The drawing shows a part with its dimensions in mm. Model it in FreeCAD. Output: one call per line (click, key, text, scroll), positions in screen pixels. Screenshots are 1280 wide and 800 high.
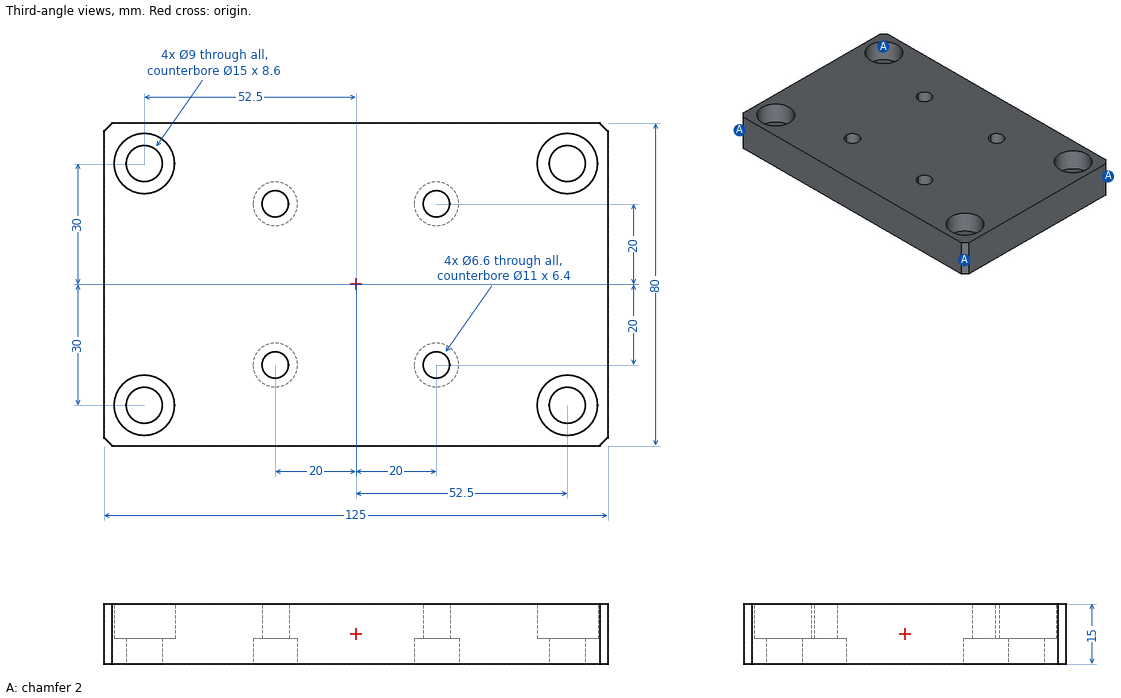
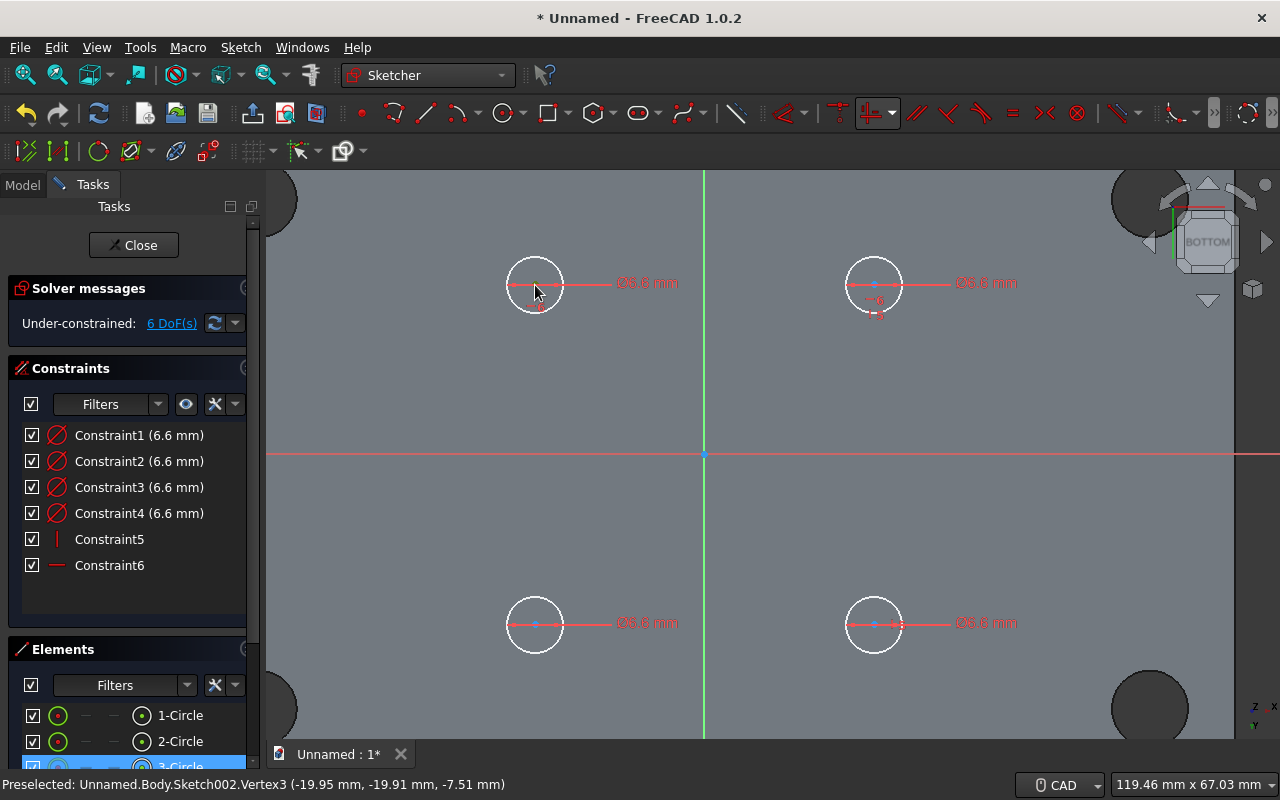
click(535, 625)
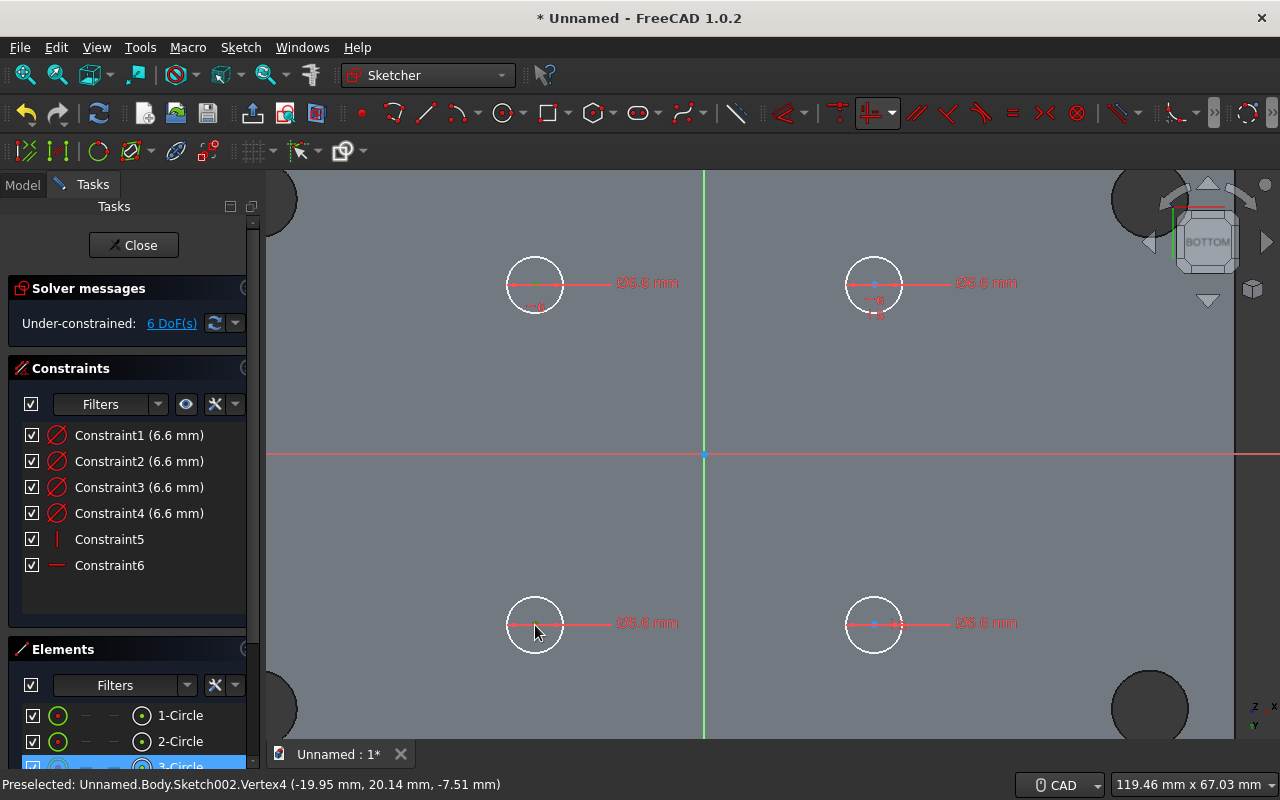
click(894, 114)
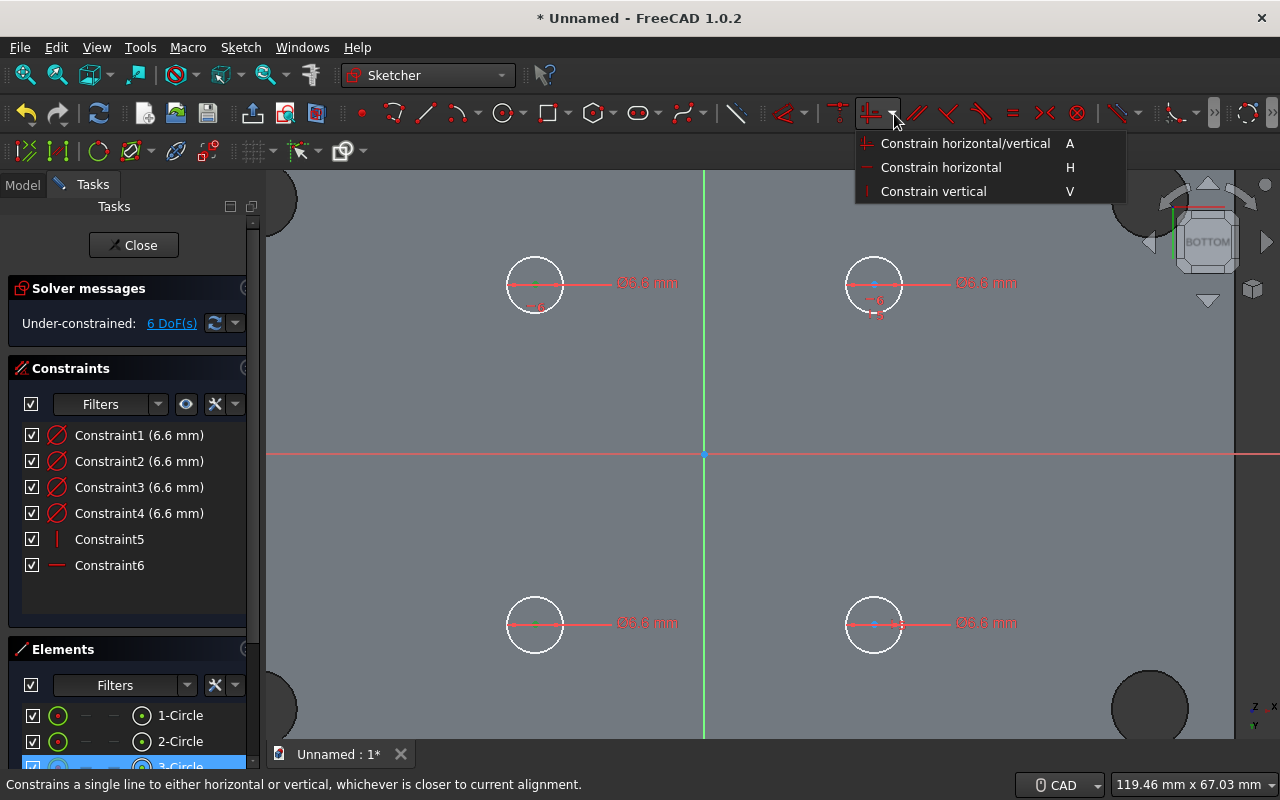
click(991, 191)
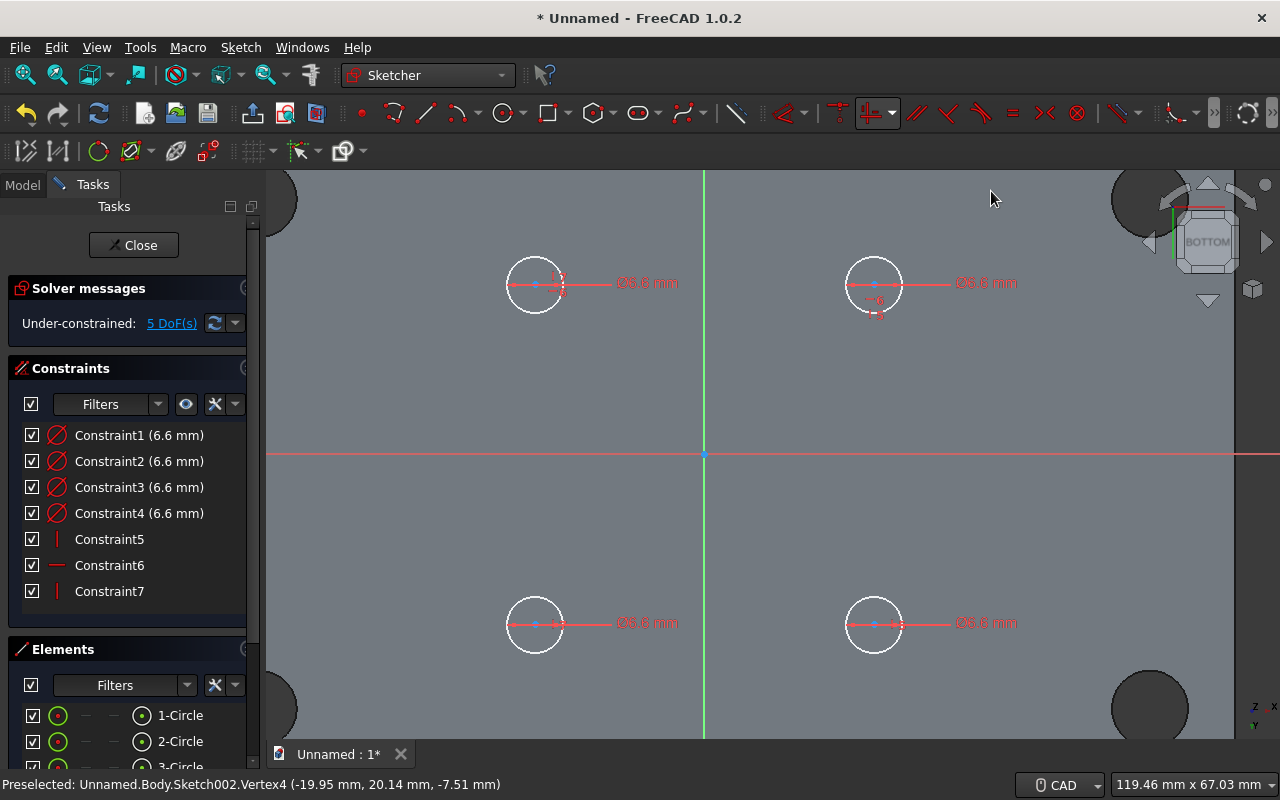
click(874, 625)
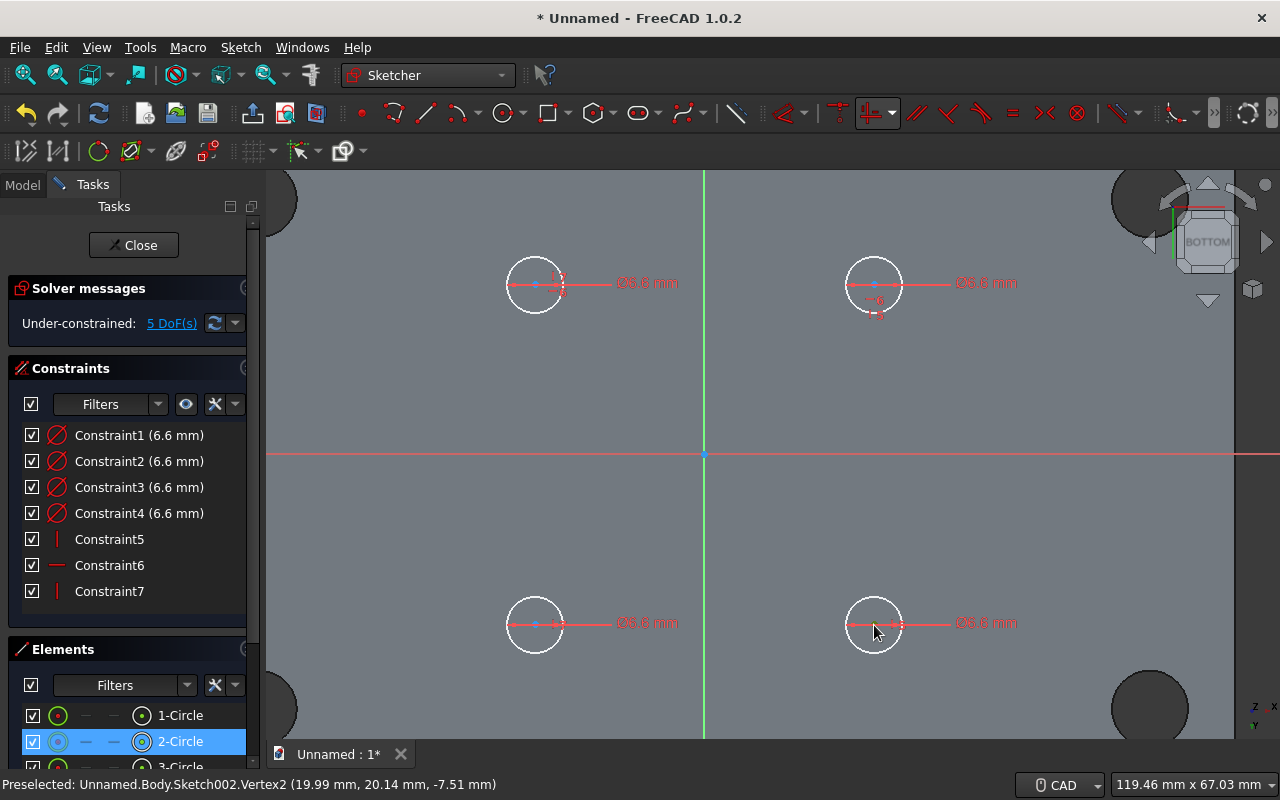
click(535, 625)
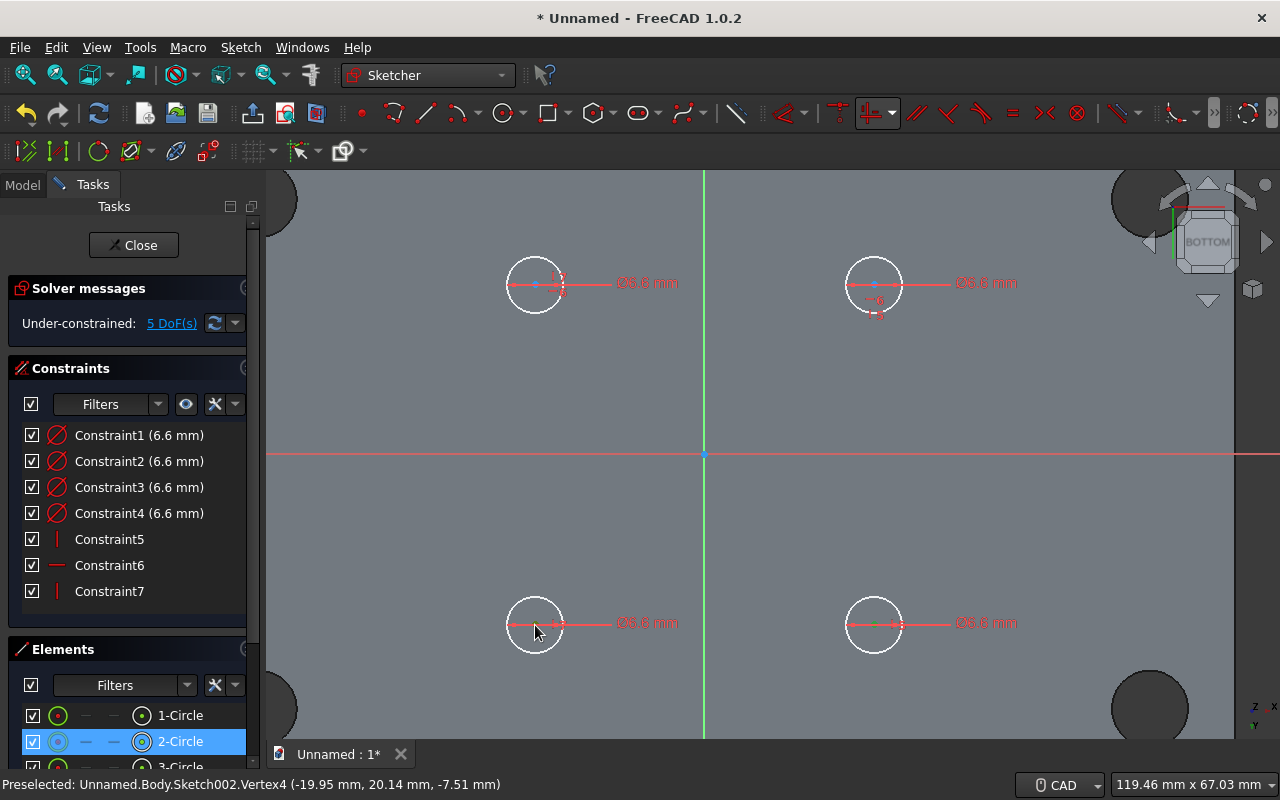
click(894, 114)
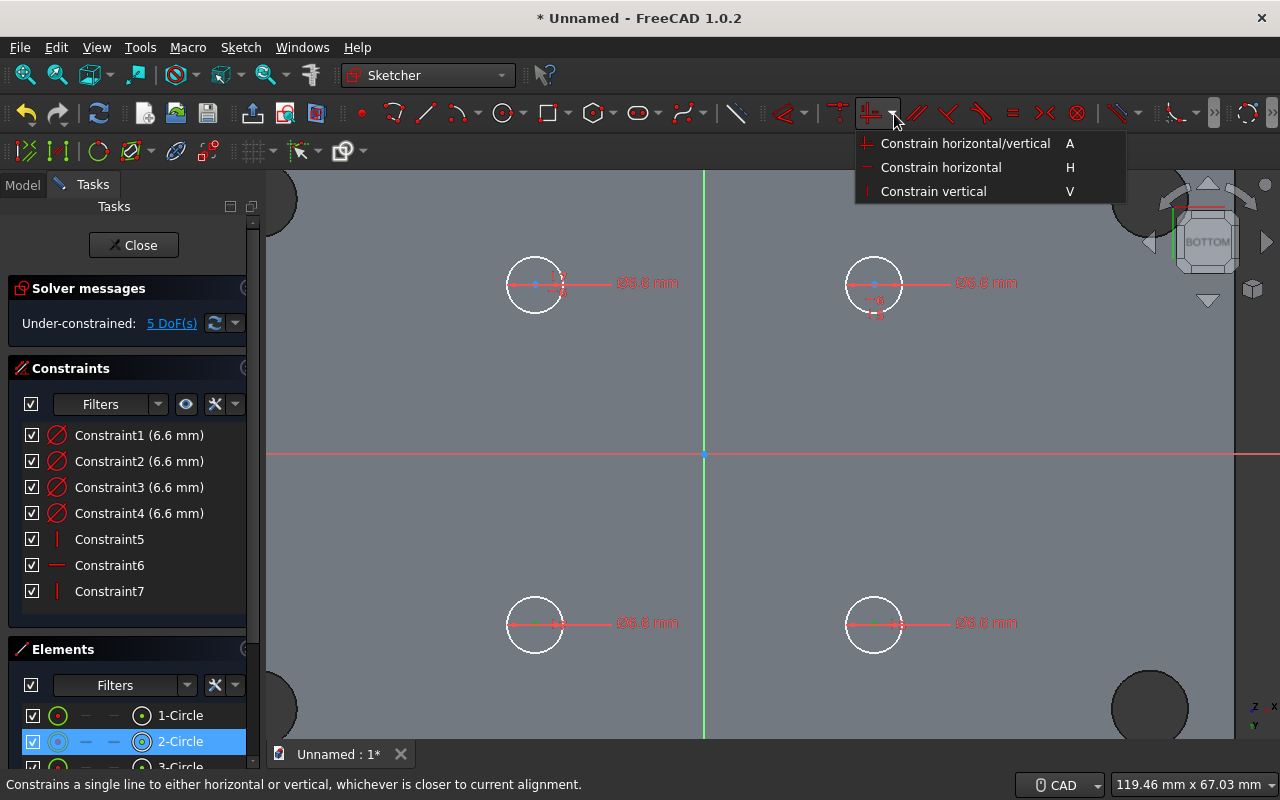
click(991, 167)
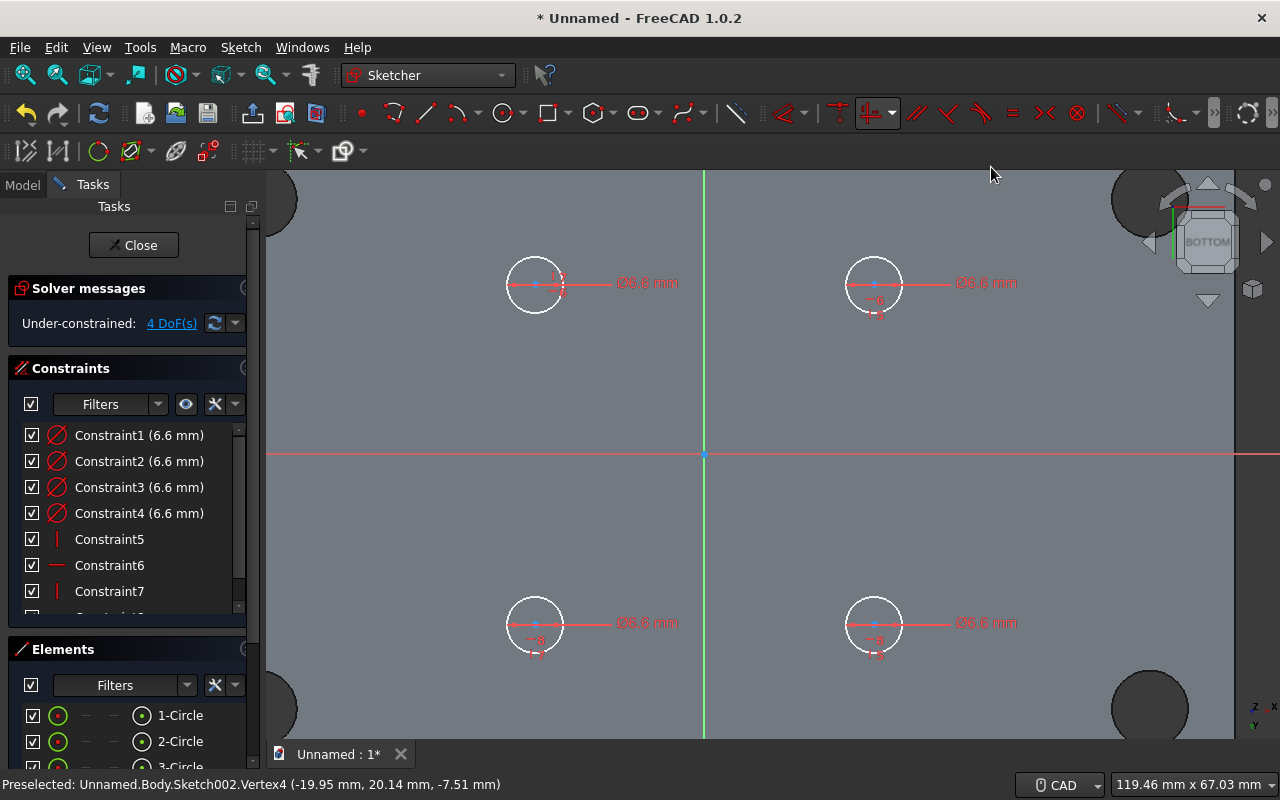
key(d)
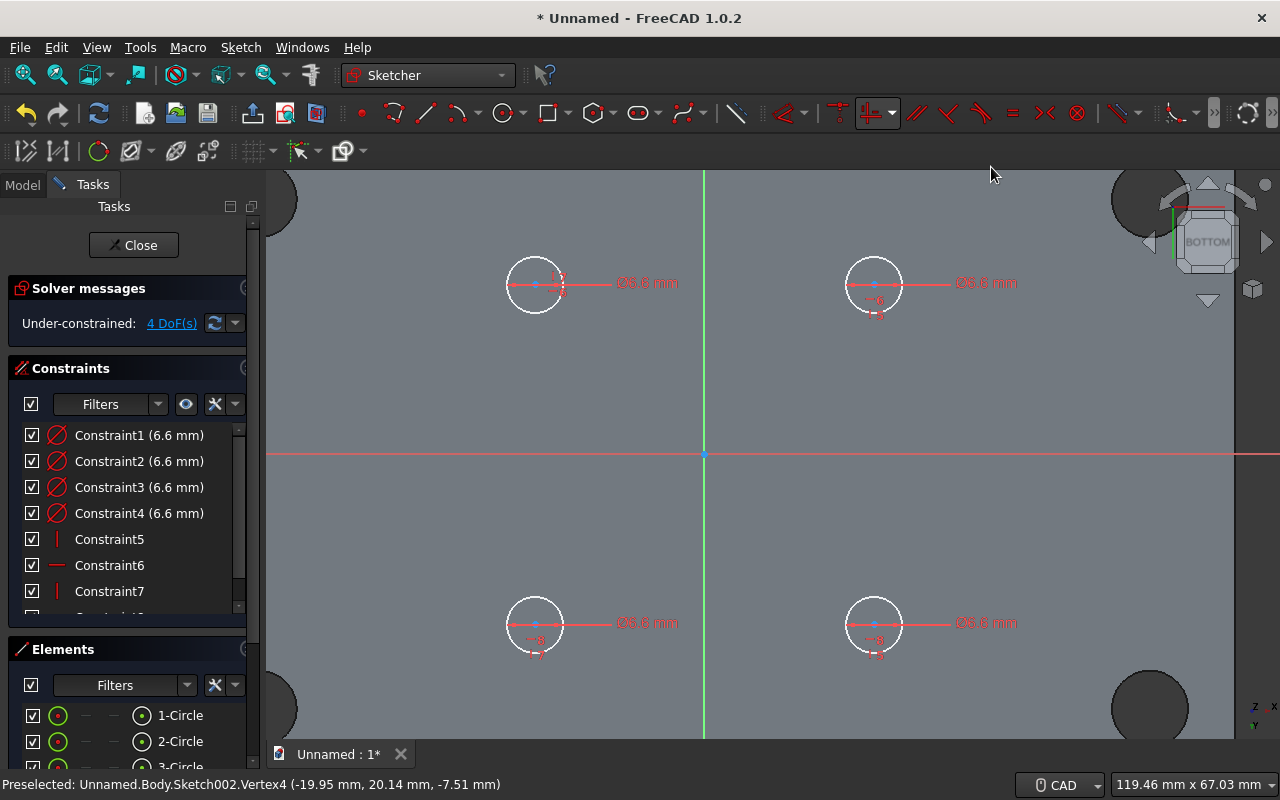
click(874, 285)
click(789, 251)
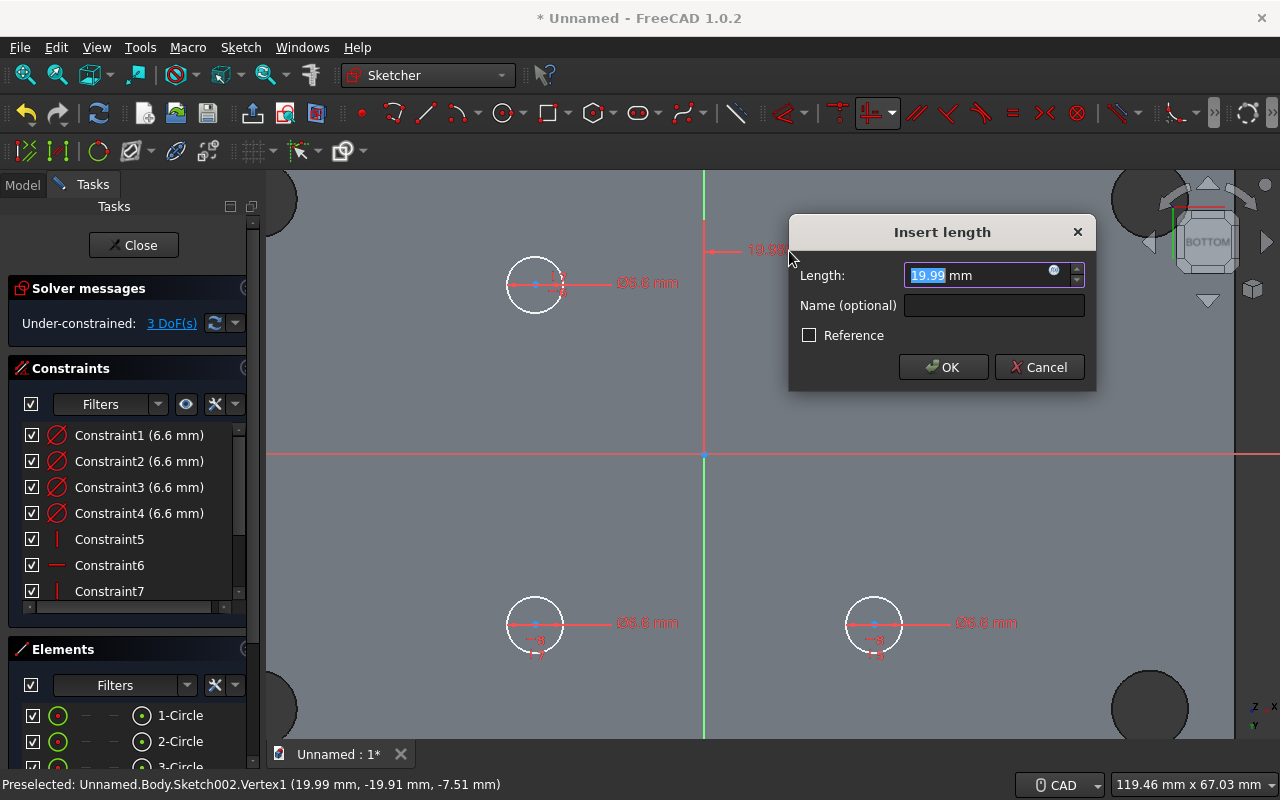
text(20)
key(Return)